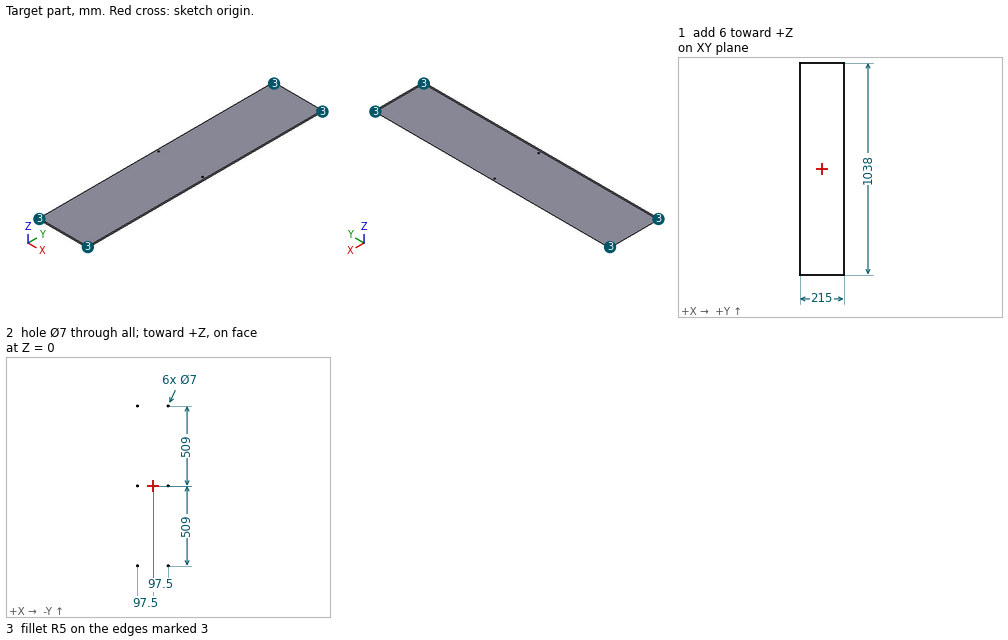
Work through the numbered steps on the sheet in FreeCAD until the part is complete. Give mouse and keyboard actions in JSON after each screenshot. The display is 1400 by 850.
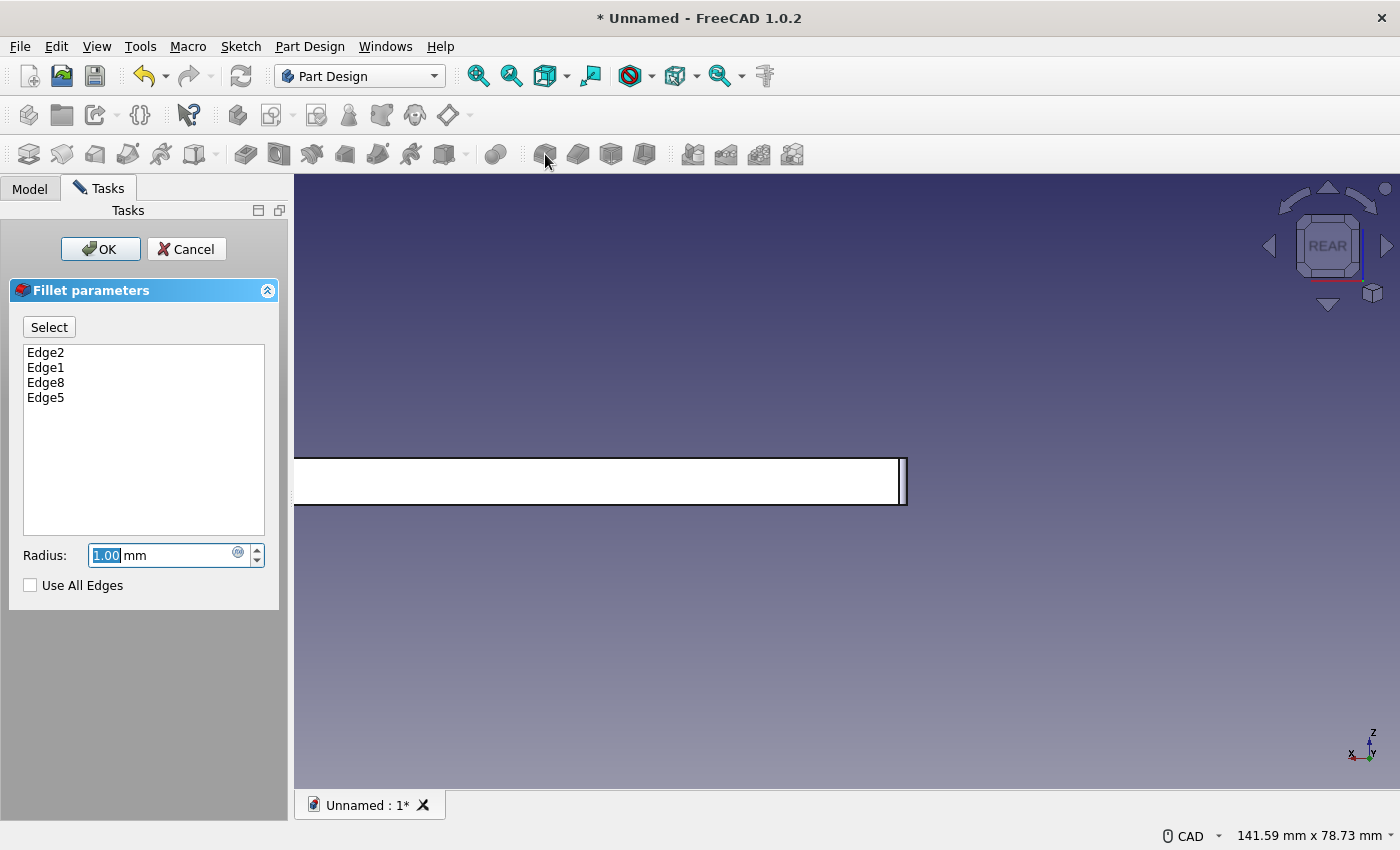
{"action": "type", "text": "5"}
{"action": "key", "text": "Tab"}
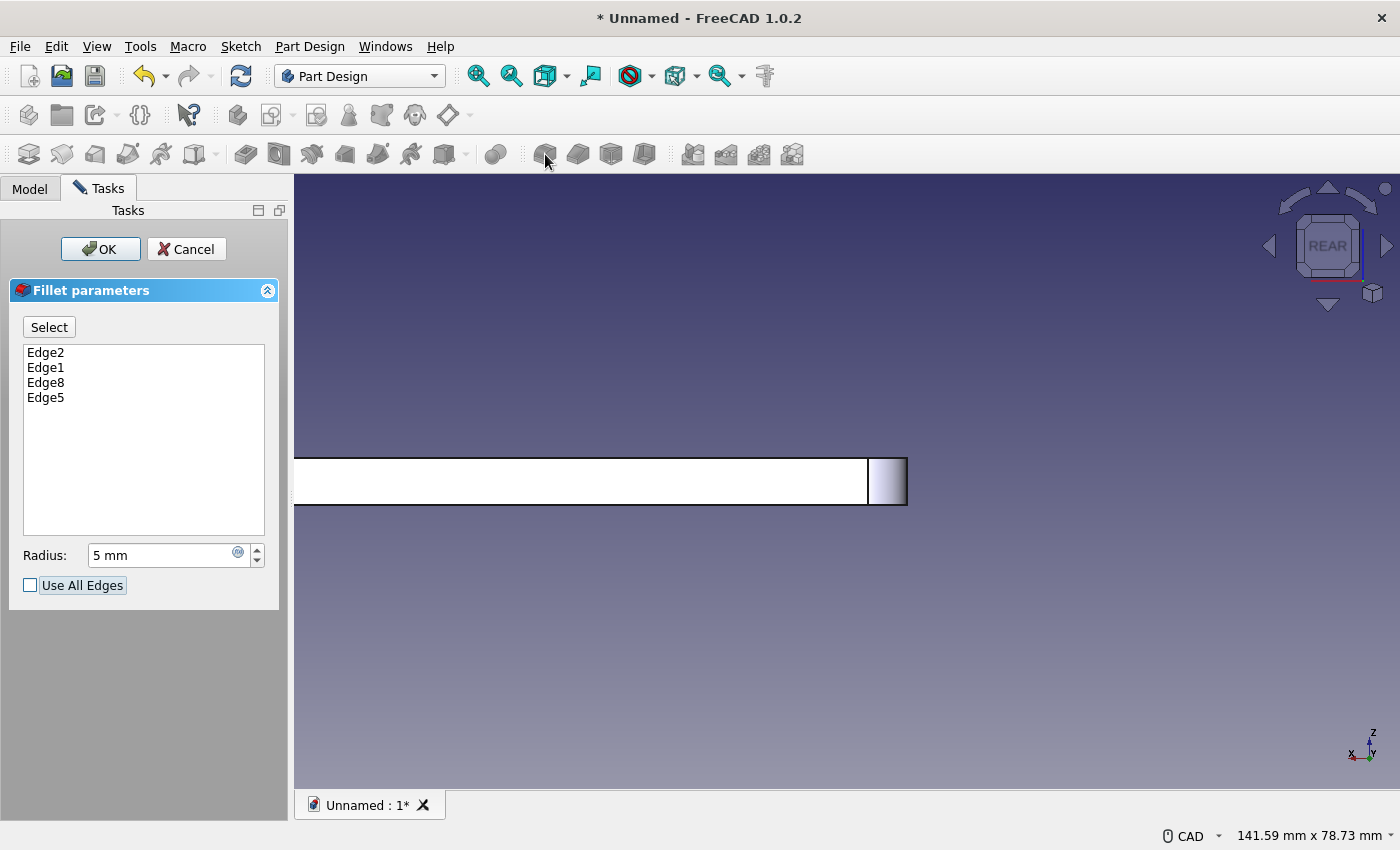
{"action": "left_click", "coordinate": [101, 249]}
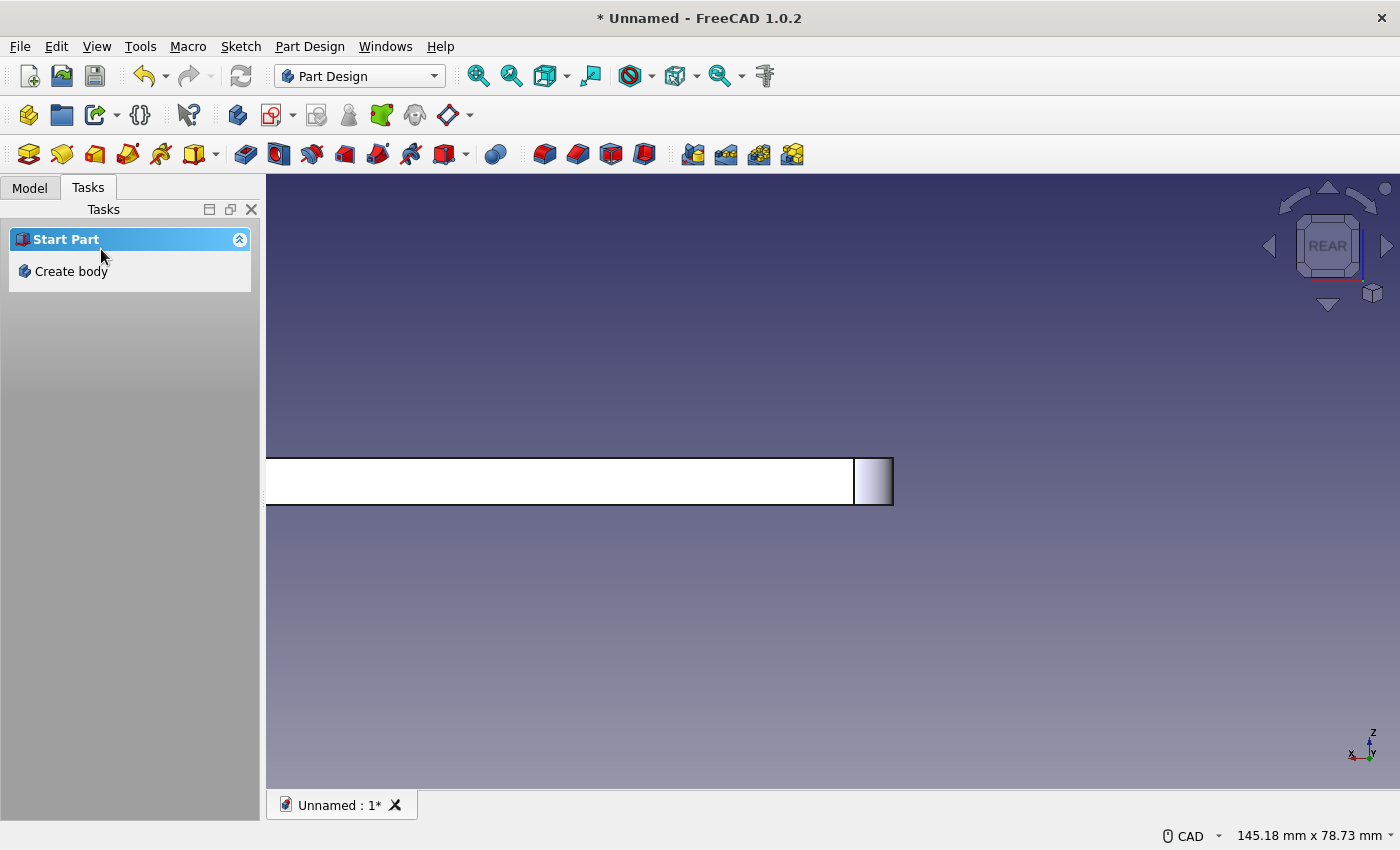
{"action": "key", "text": "0"}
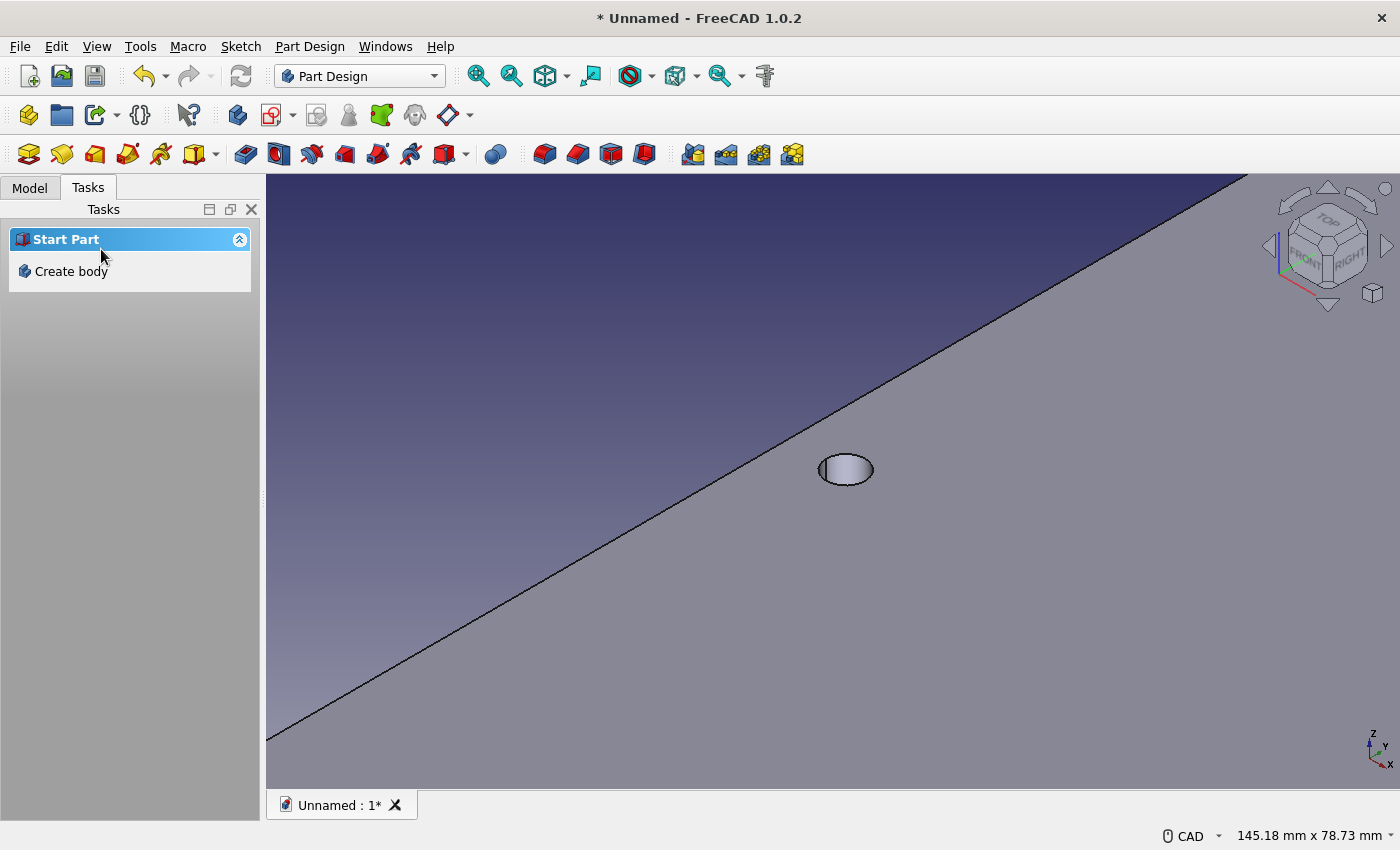
{"action": "left_click", "coordinate": [479, 76]}